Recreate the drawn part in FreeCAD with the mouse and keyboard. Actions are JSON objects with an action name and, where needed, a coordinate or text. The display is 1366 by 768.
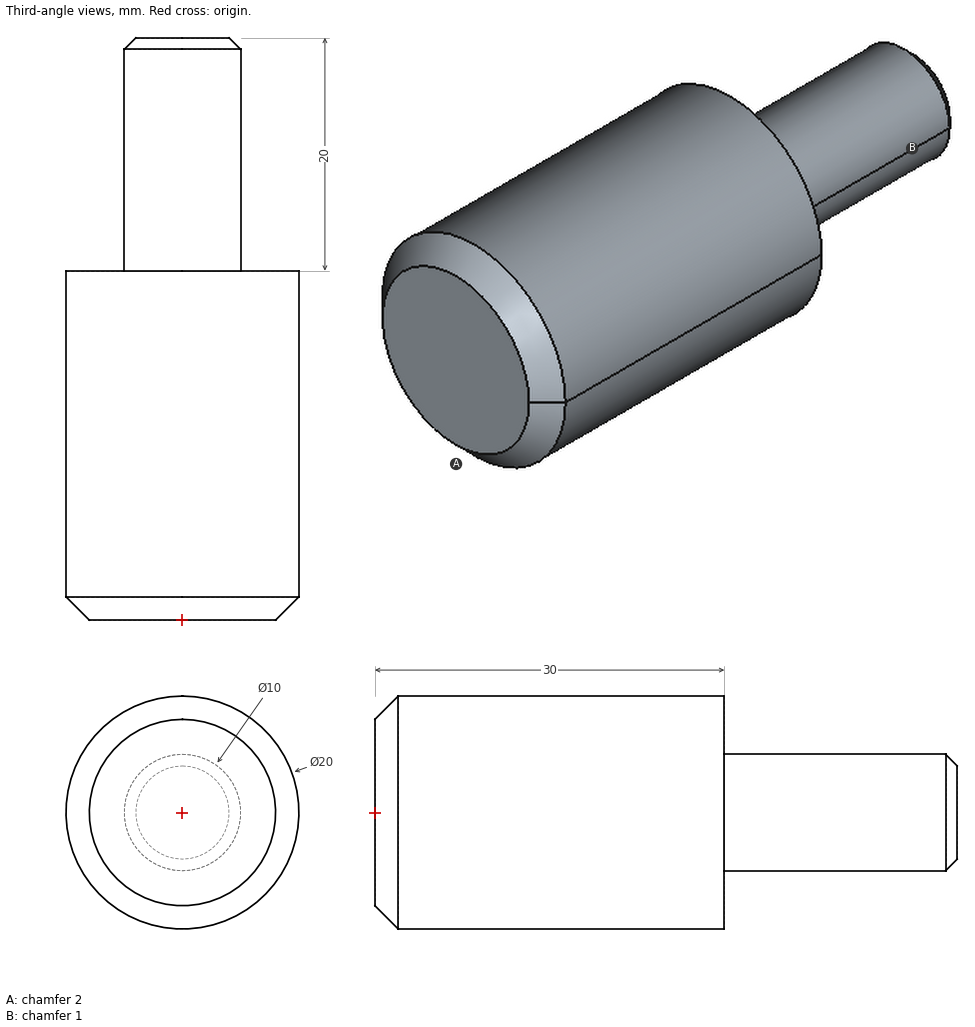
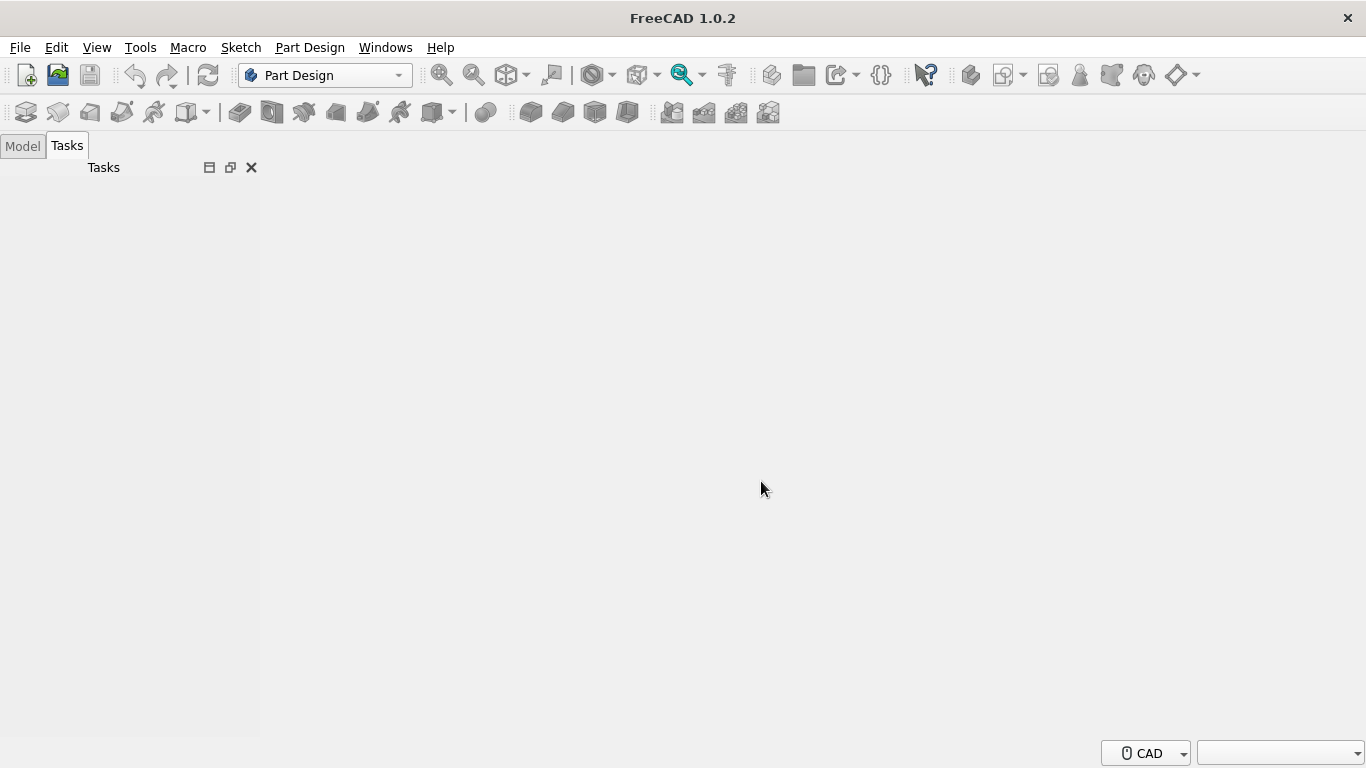
{"action": "left_click", "coordinate": [26, 76]}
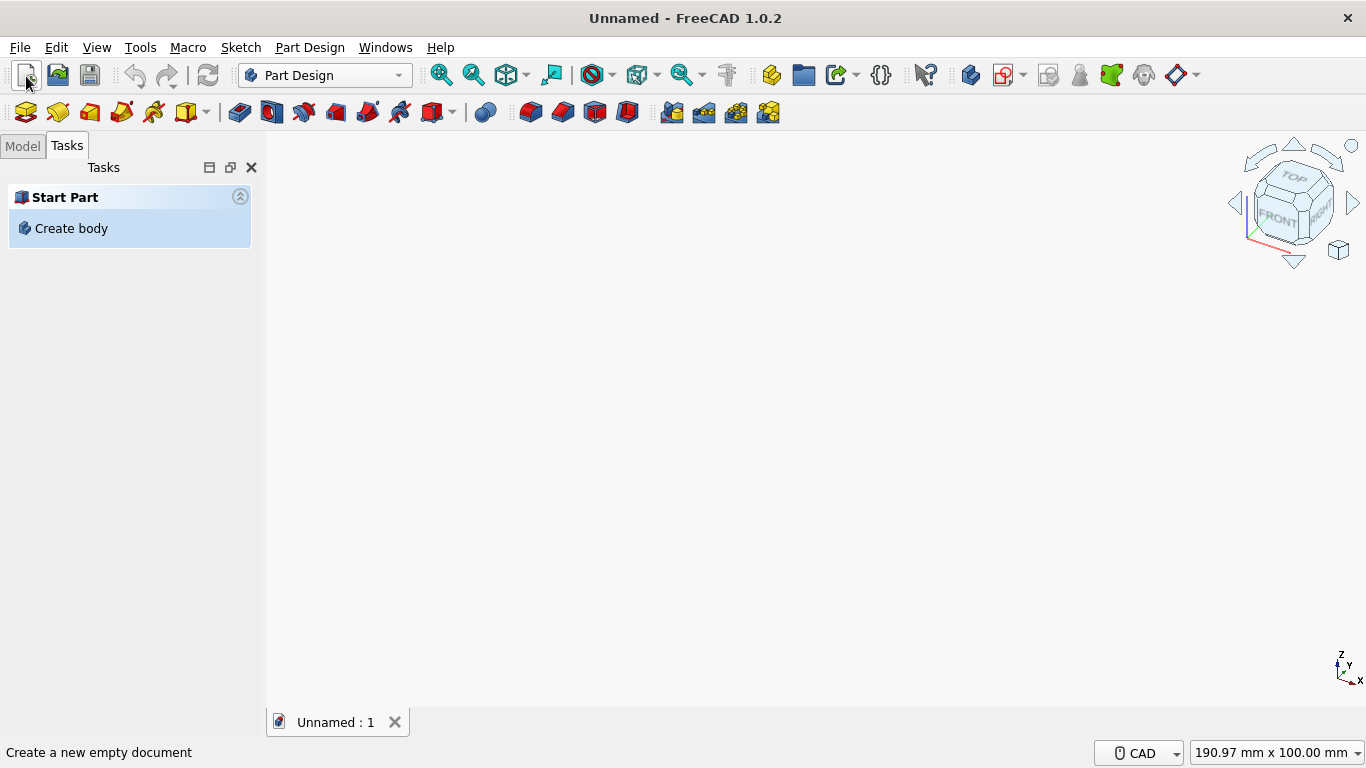
{"action": "left_click", "coordinate": [1004, 76]}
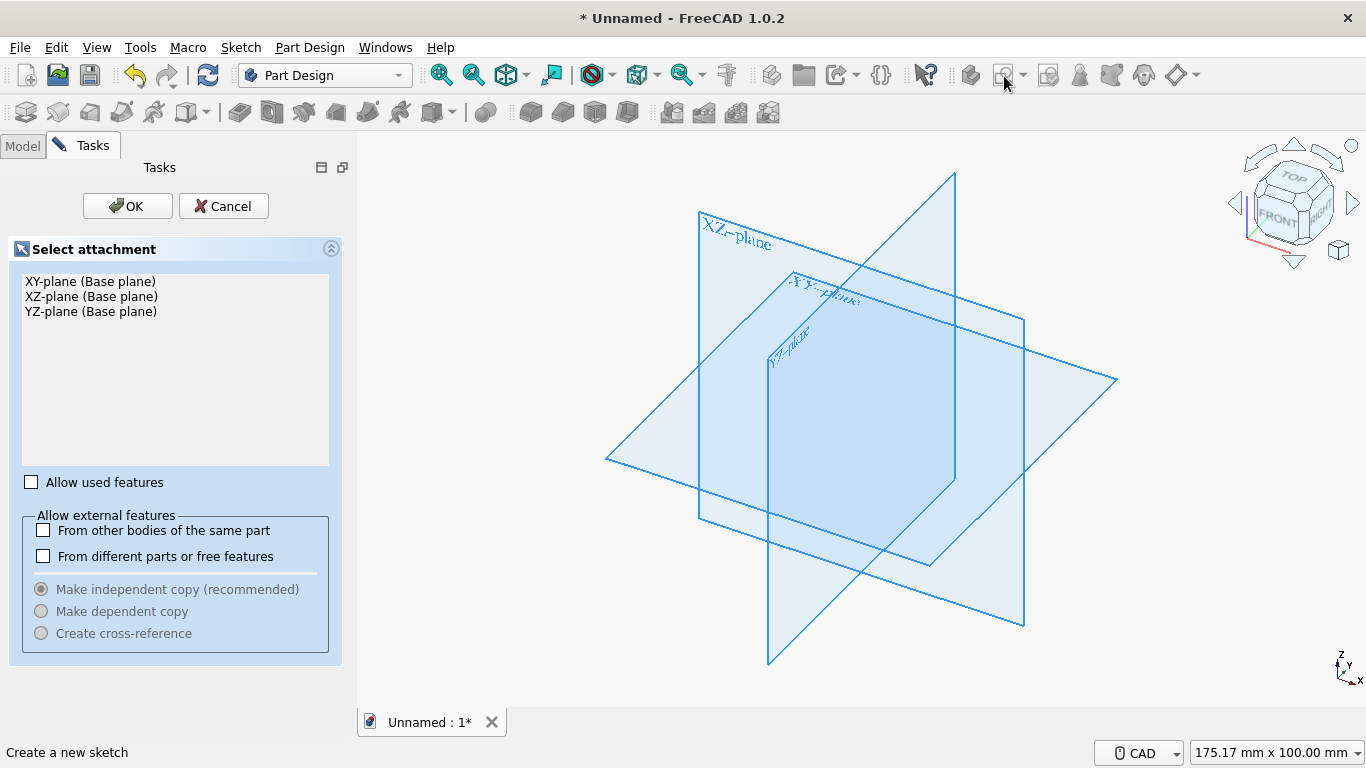
{"action": "left_click", "coordinate": [82, 296]}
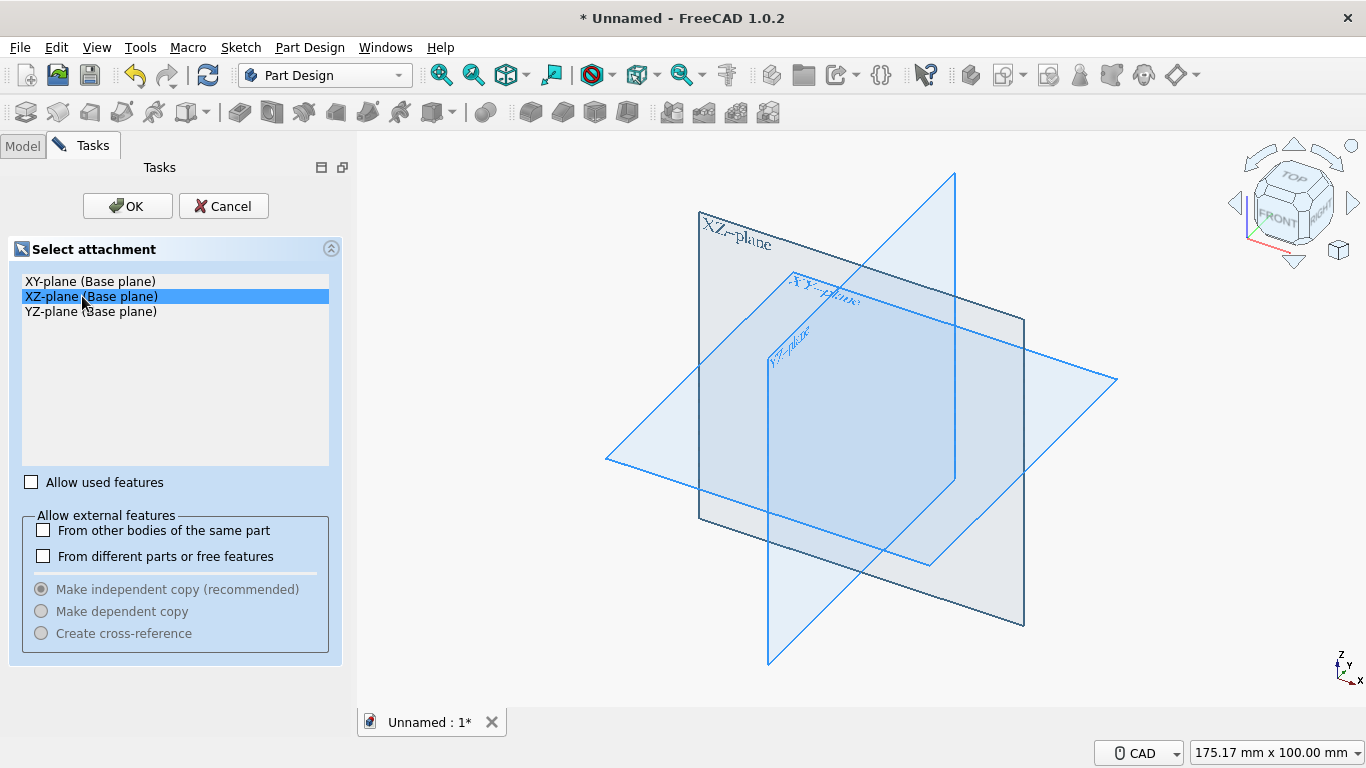
{"action": "left_click", "coordinate": [128, 206]}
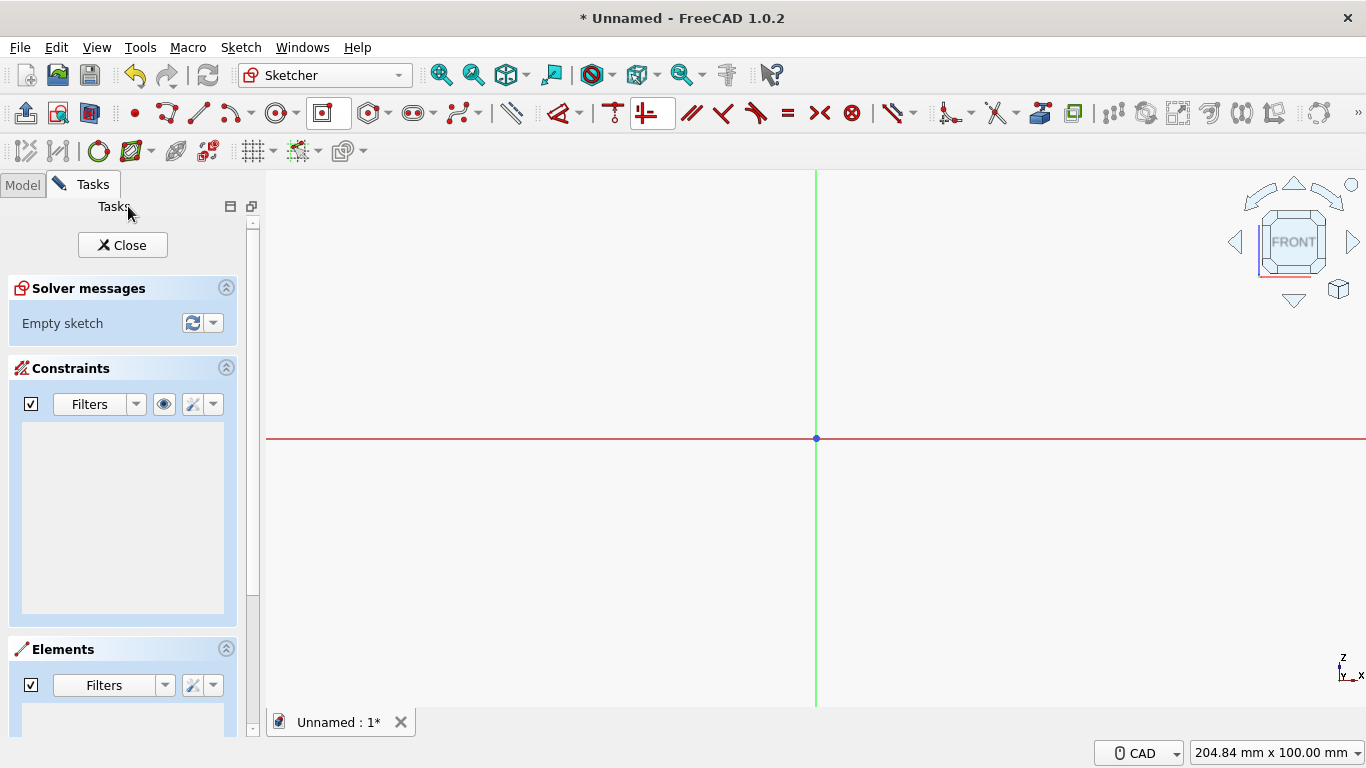
{"action": "scroll", "coordinate": [846, 438], "scroll_direction": "up", "scroll_amount": 6}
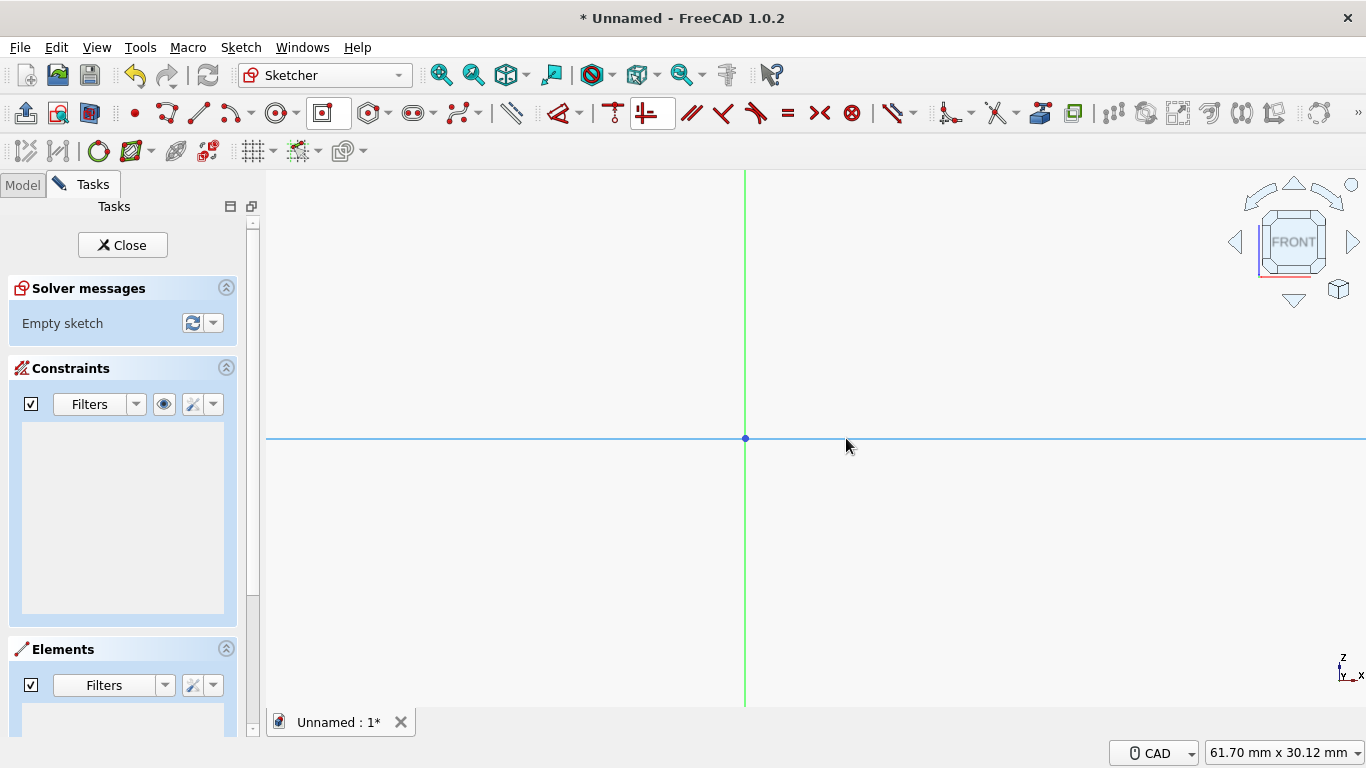
{"action": "left_click", "coordinate": [276, 114]}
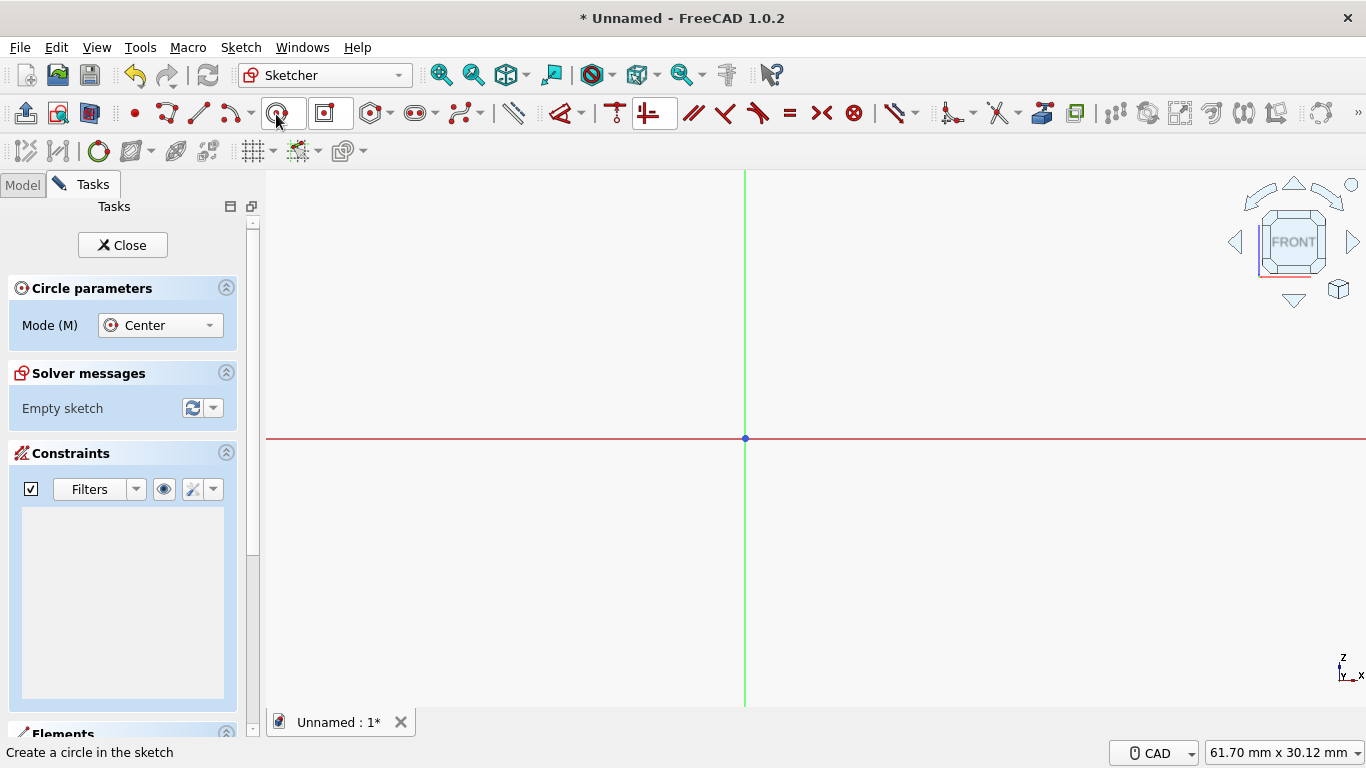
{"action": "left_click", "coordinate": [745, 438]}
{"action": "mouse_move", "coordinate": [871, 312]}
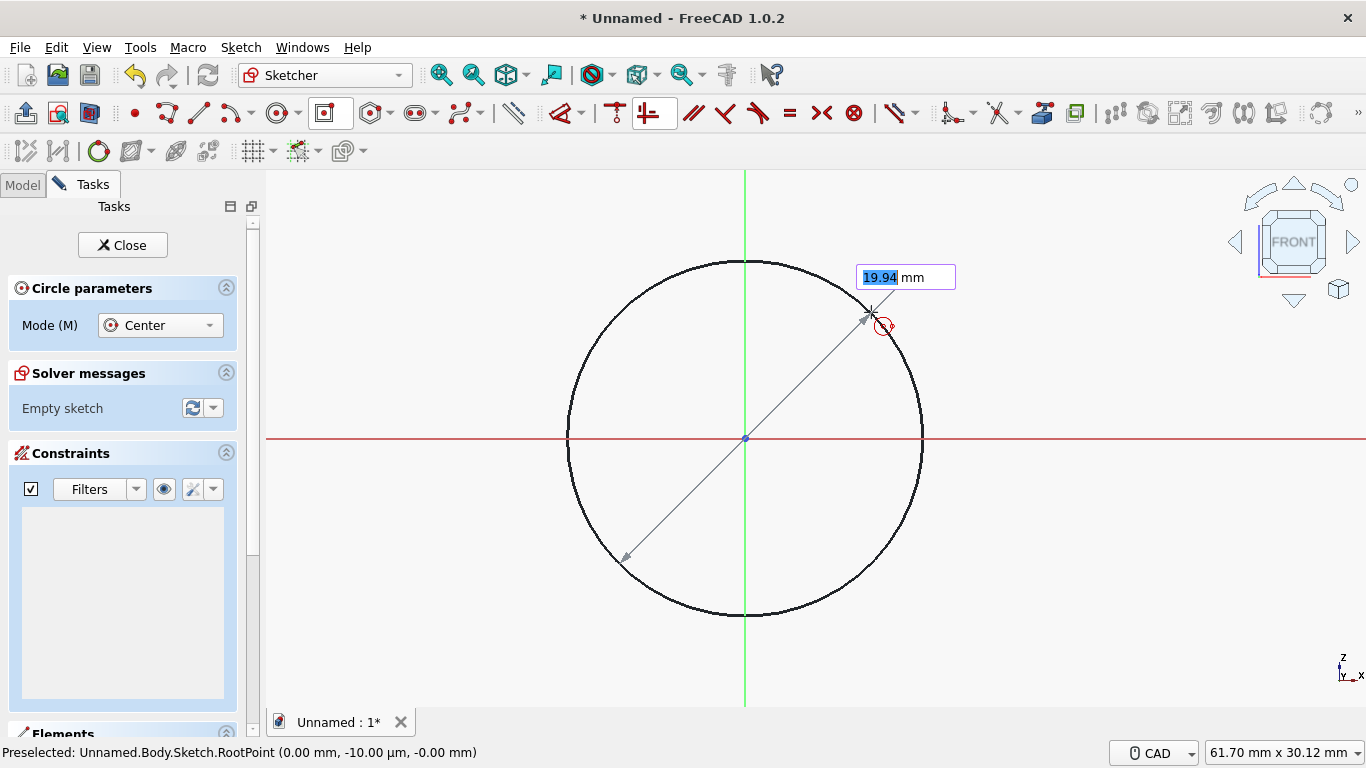
{"action": "type", "text": "20"}
{"action": "key", "text": "Return"}
{"action": "key", "text": "Escape"}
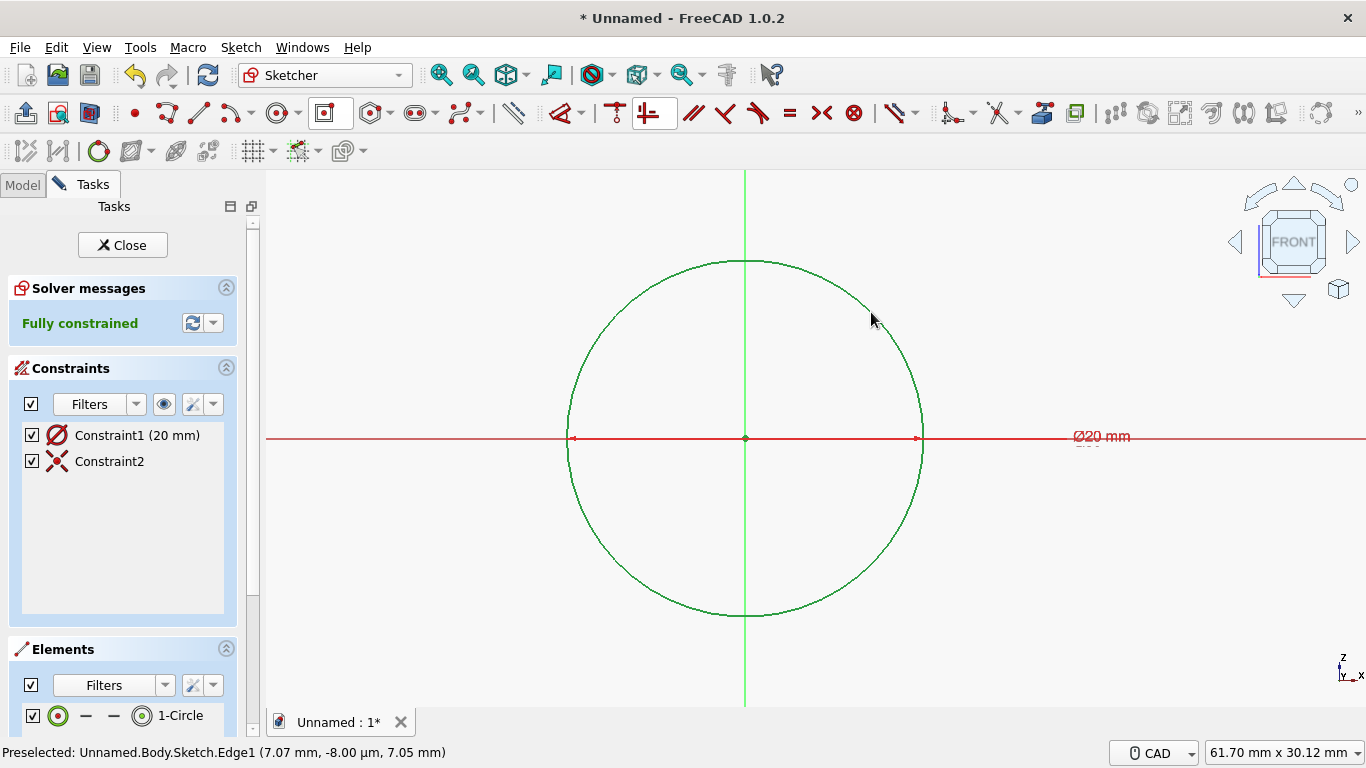
{"action": "left_click", "coordinate": [123, 245]}